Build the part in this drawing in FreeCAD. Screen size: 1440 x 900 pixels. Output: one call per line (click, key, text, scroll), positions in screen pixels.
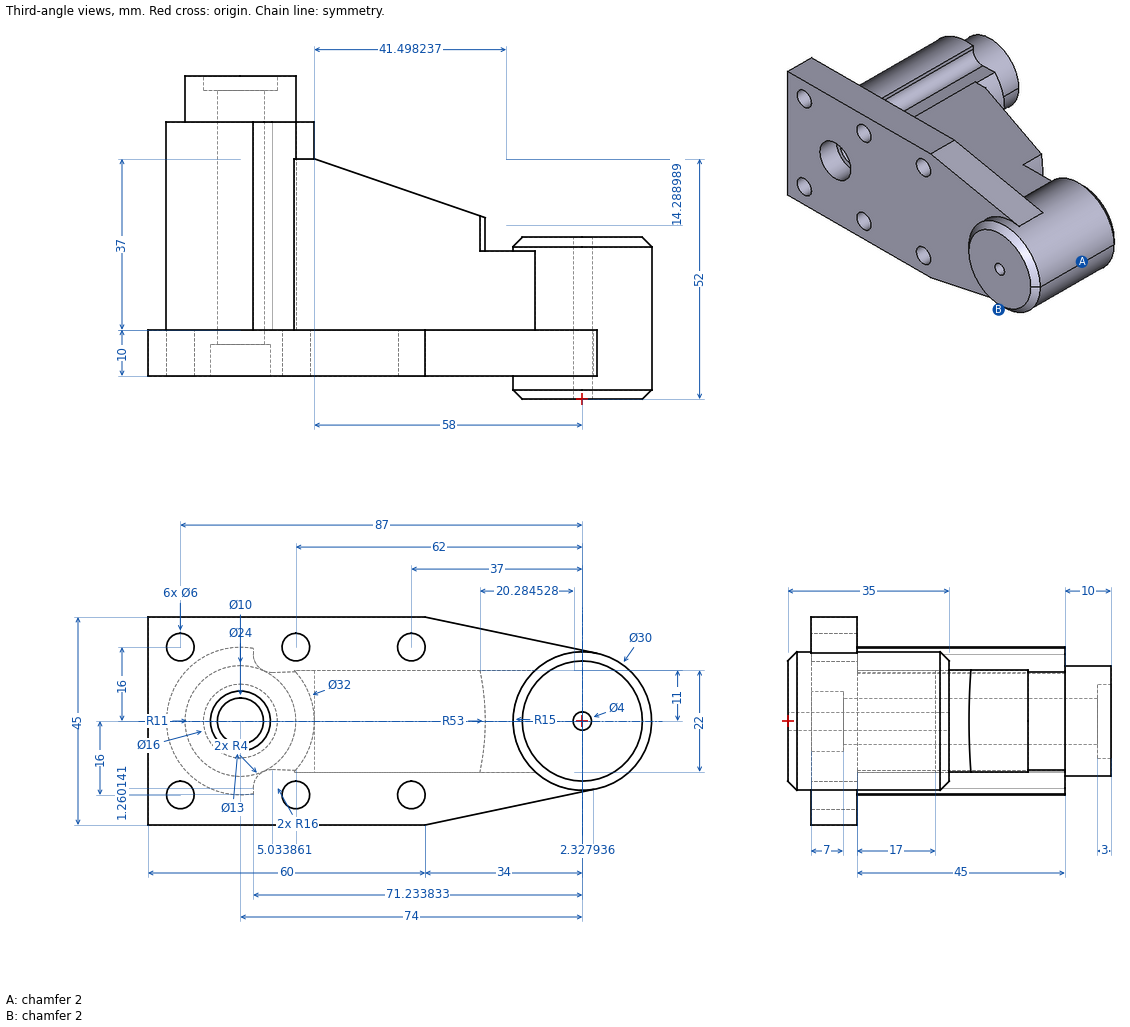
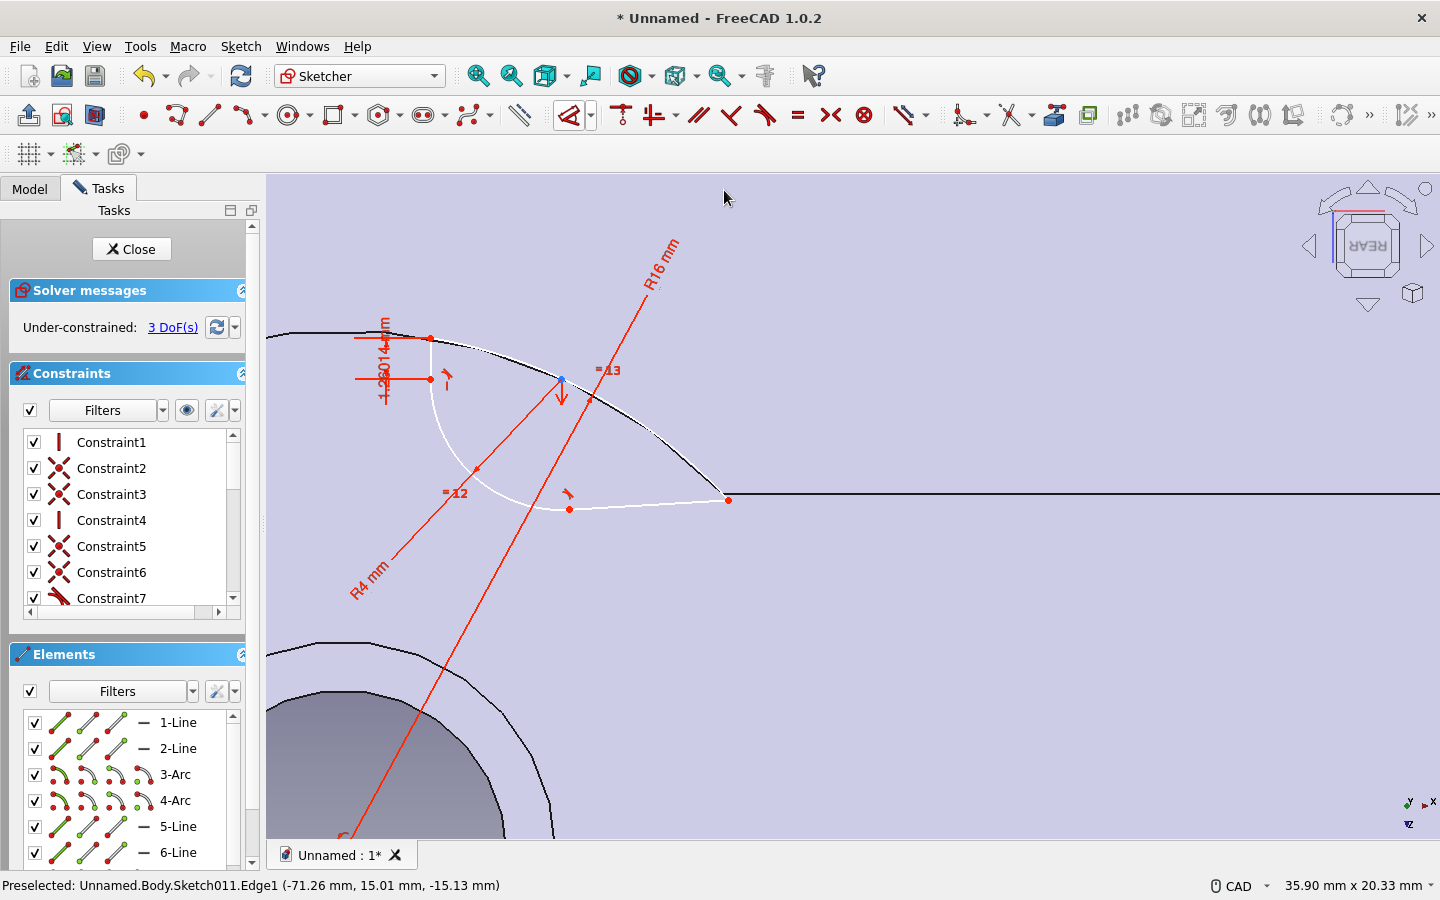
click(617, 507)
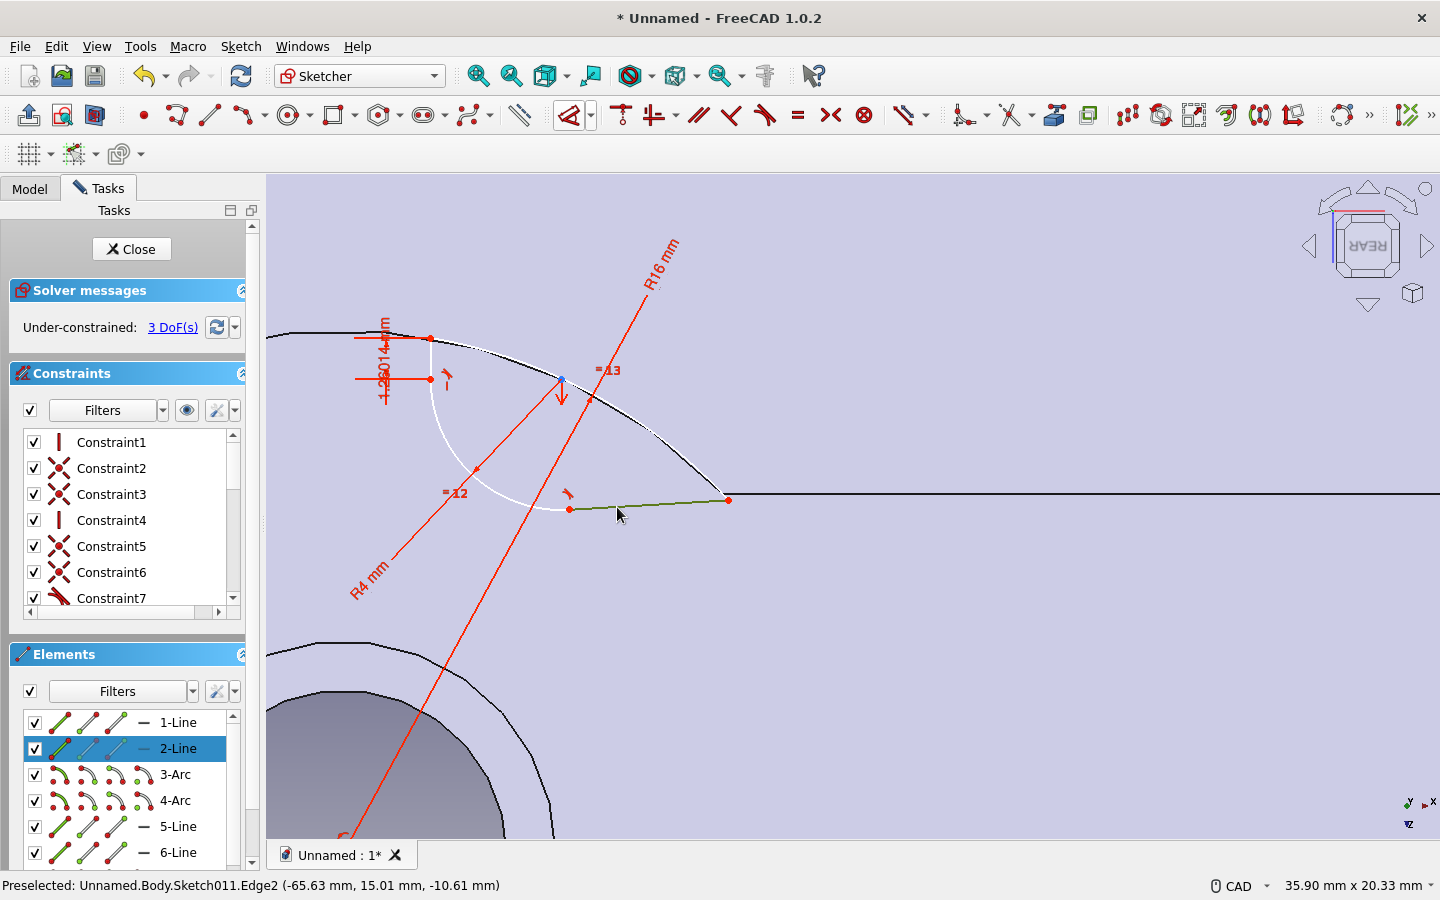
key(l)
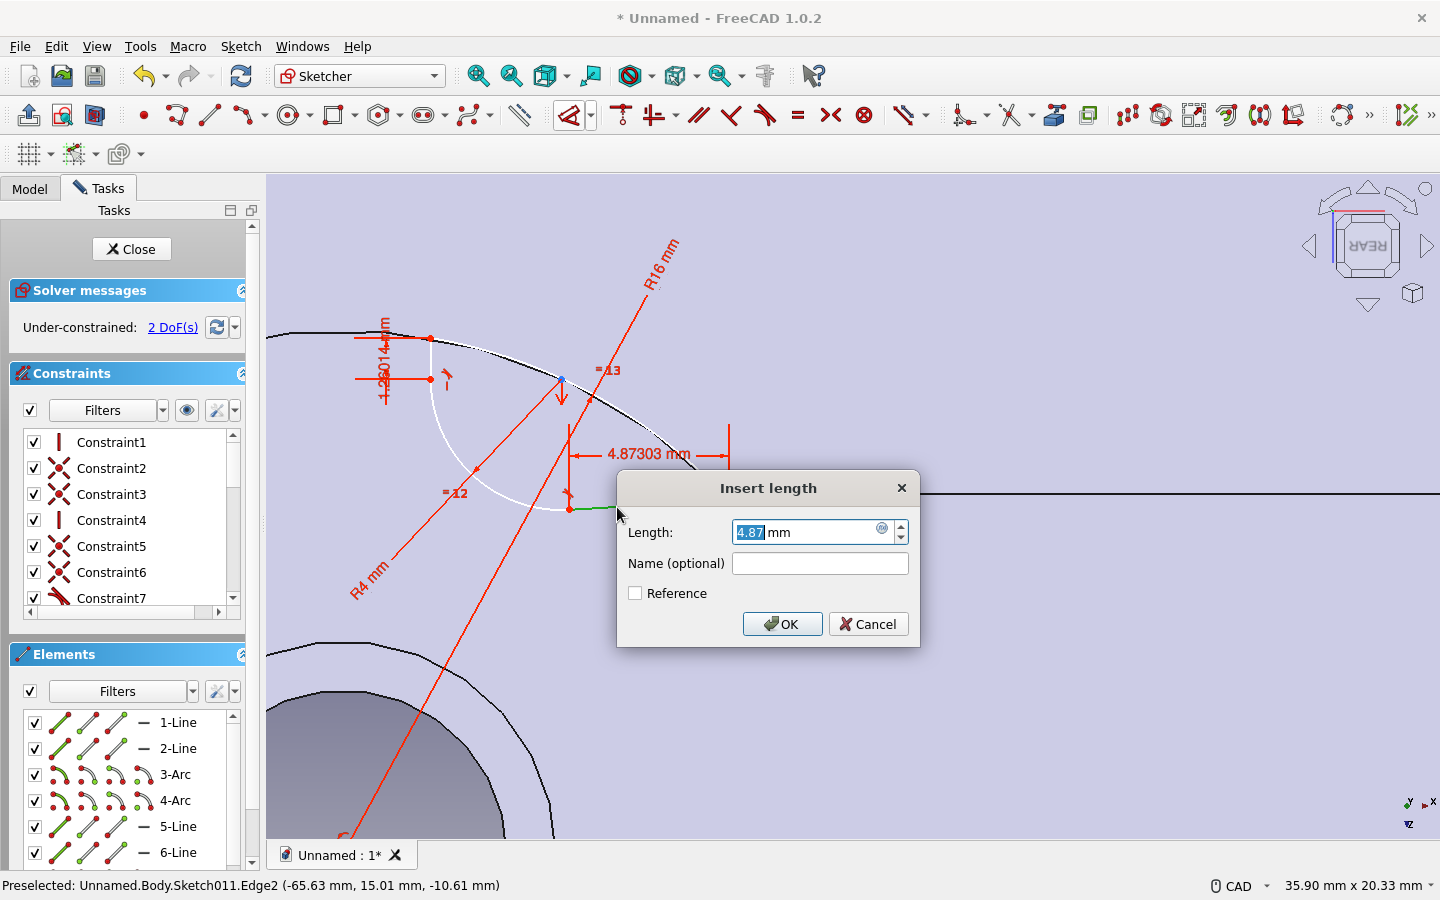
text(5.033861)
key(Return)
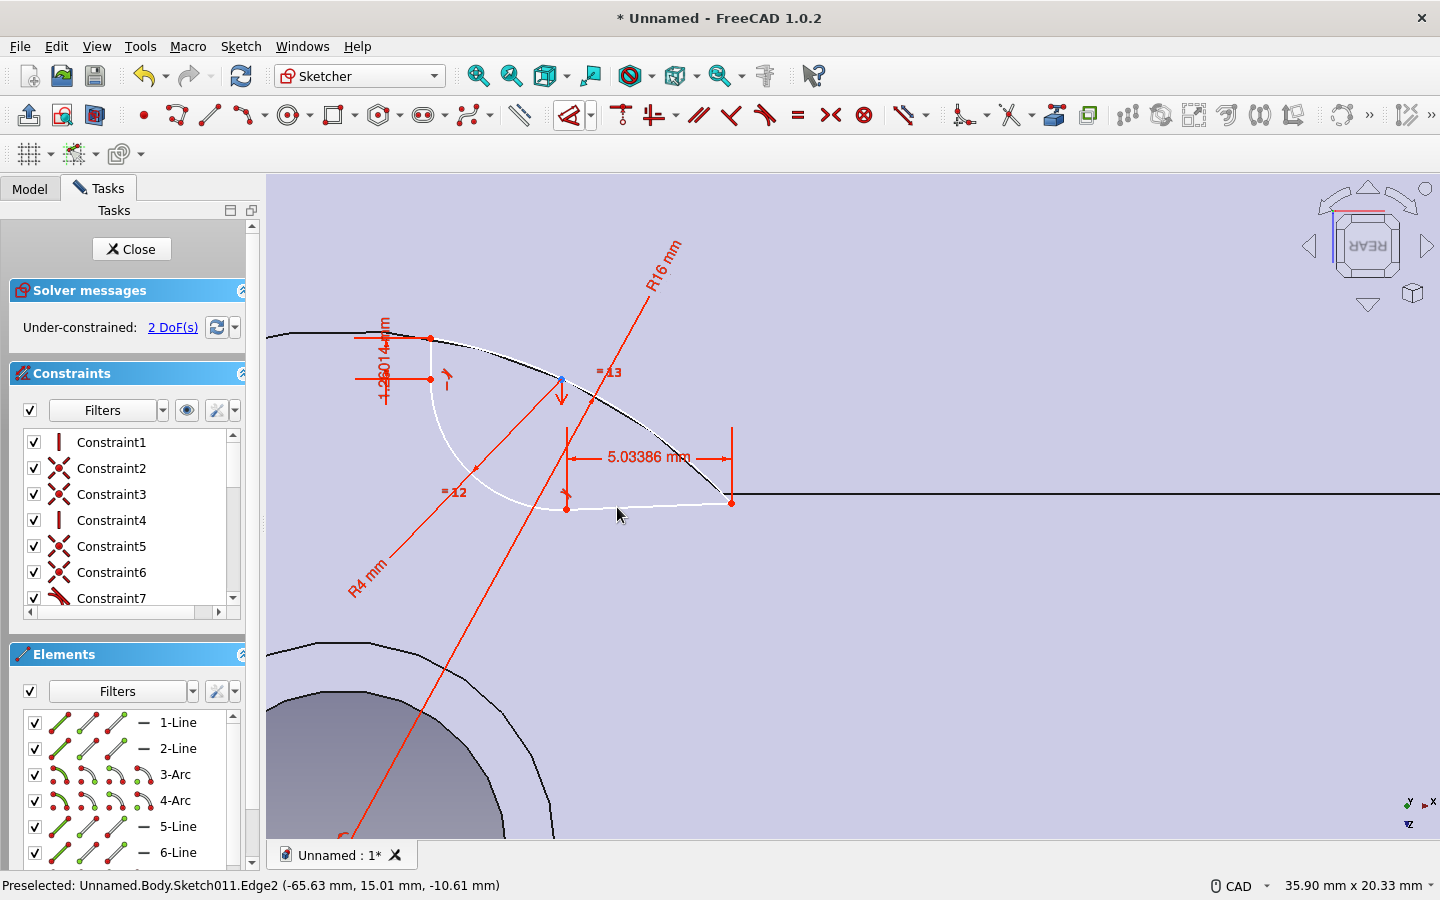
scroll(434, 357, down, 6)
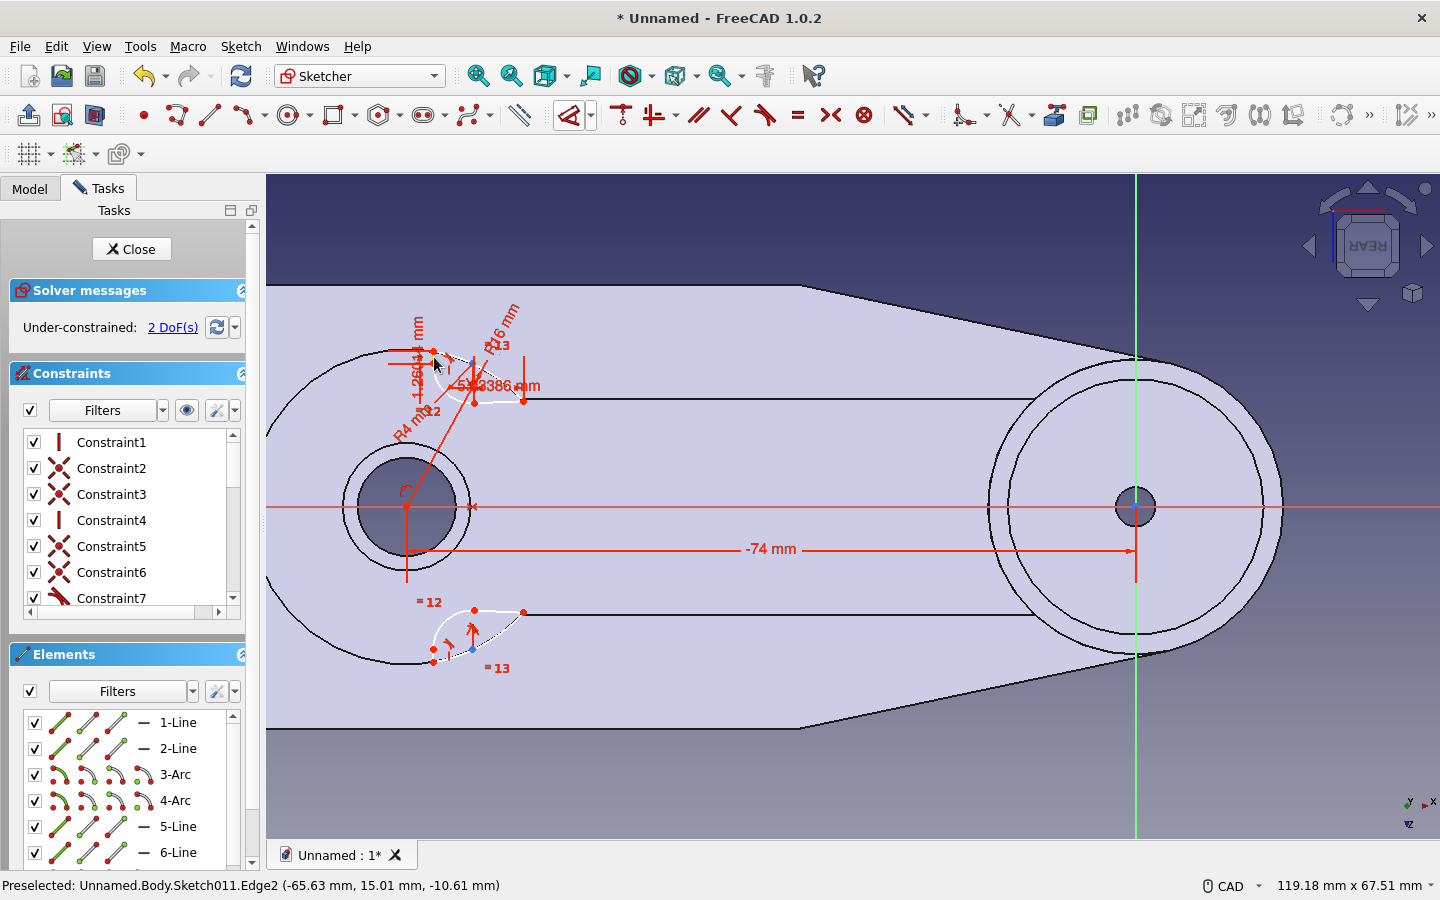
scroll(509, 612, up, 2)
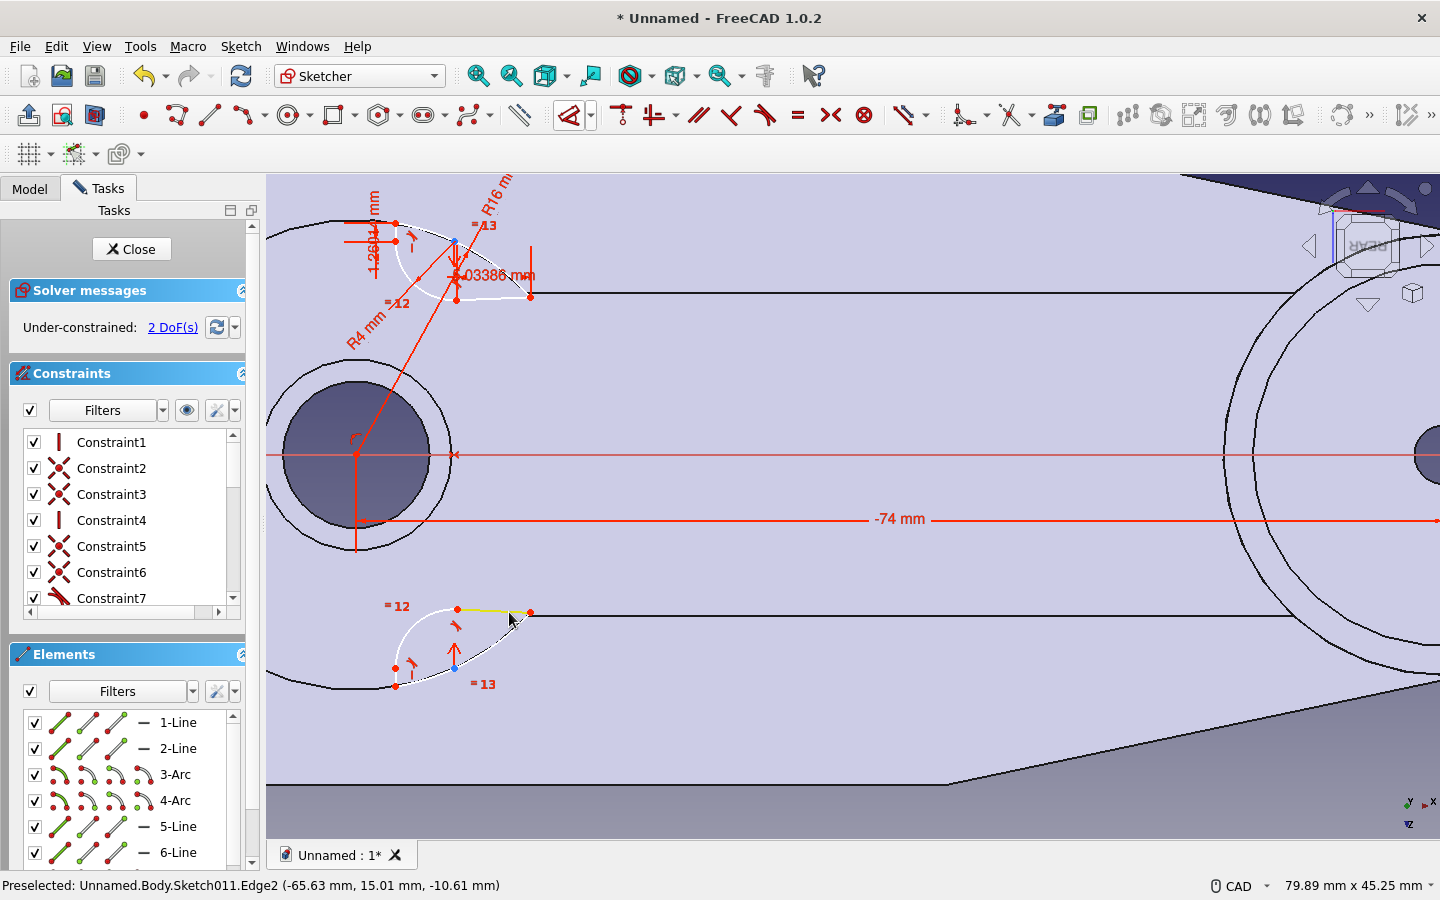
click(508, 612)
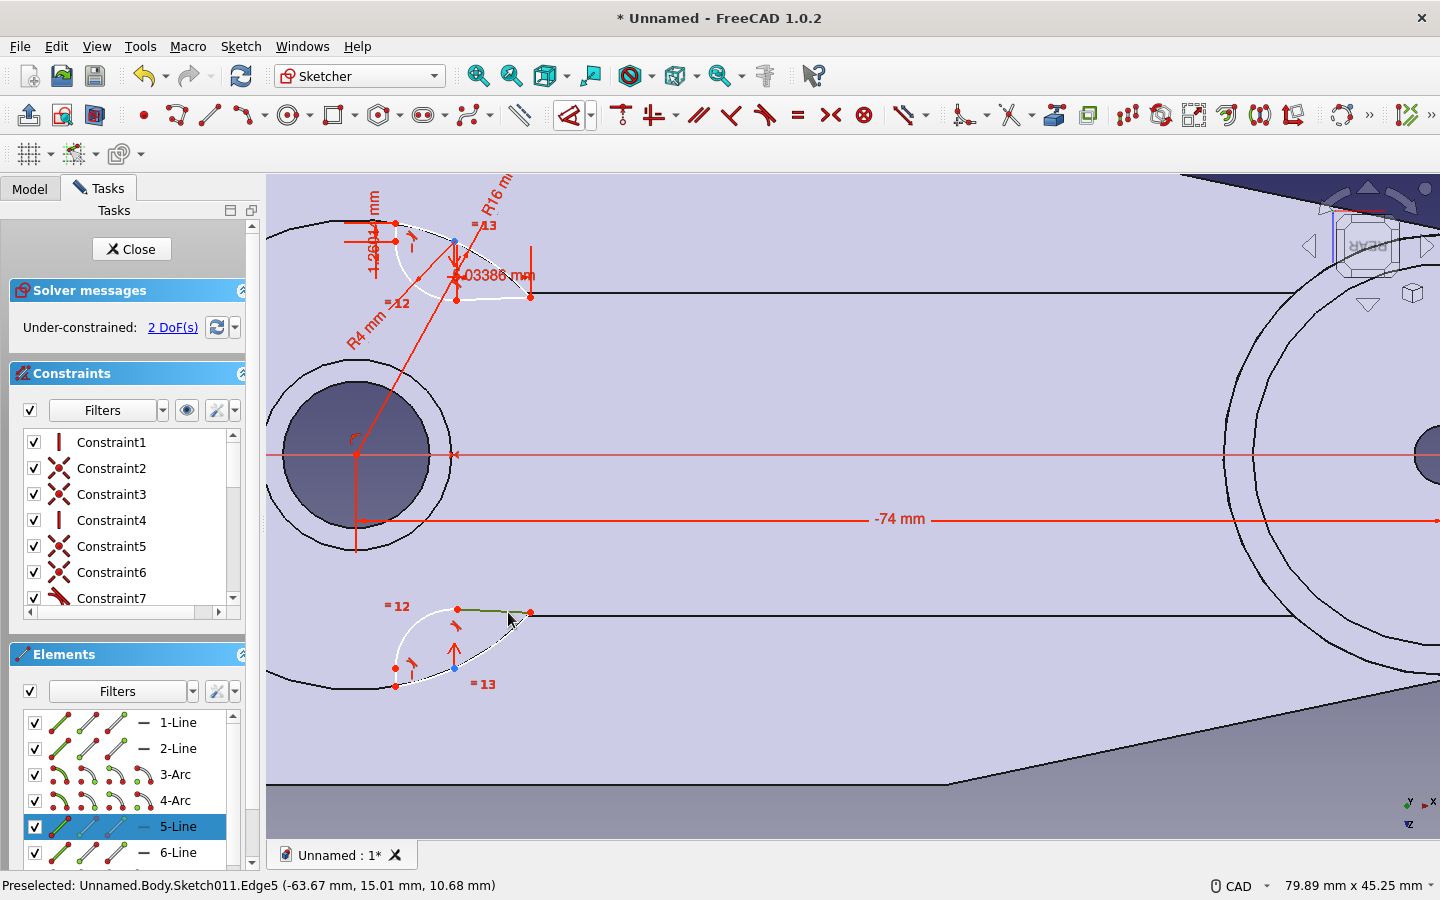
click(590, 116)